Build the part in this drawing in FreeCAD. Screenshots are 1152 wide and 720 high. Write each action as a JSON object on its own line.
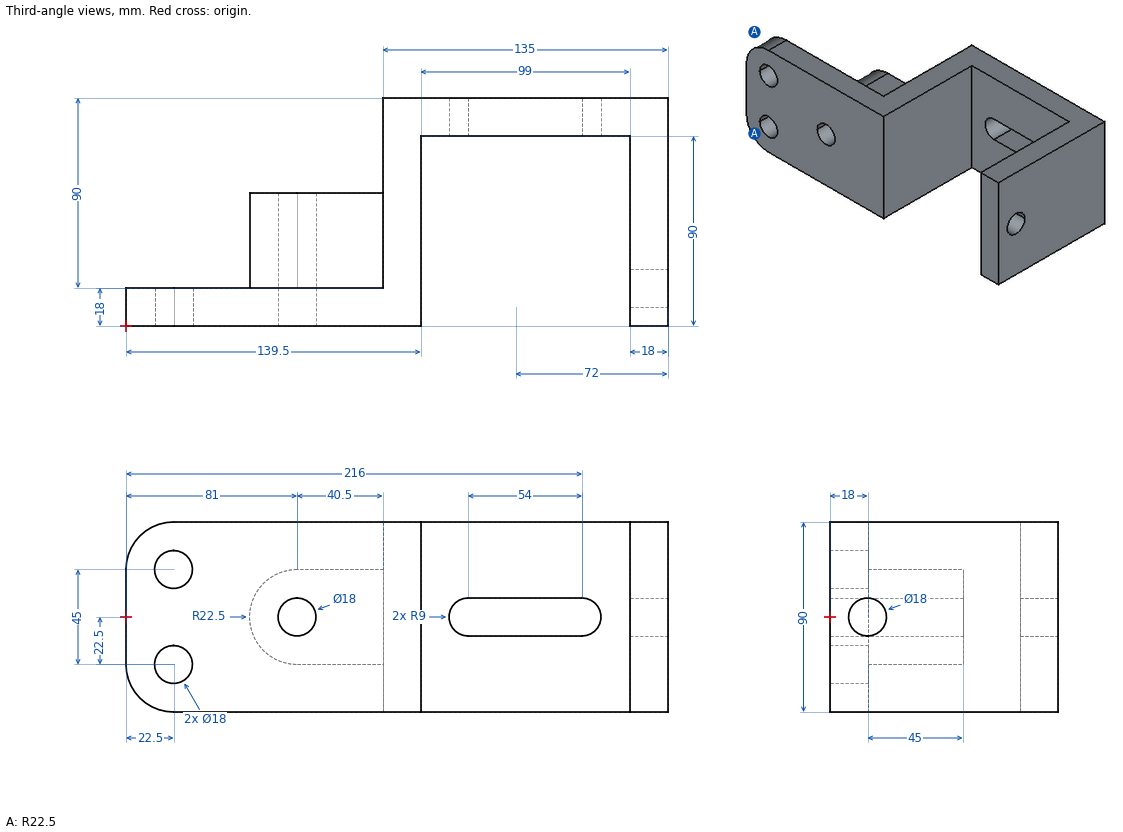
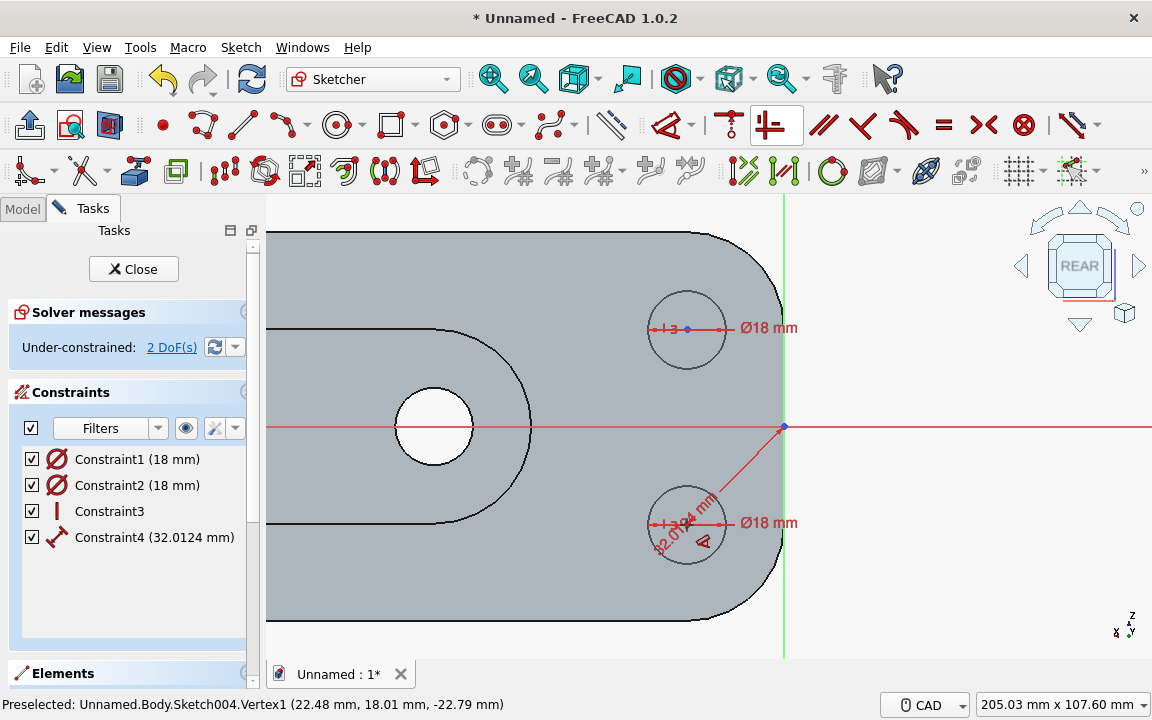
{"action": "left_click", "coordinate": [687, 330]}
{"action": "left_click", "coordinate": [653, 383]}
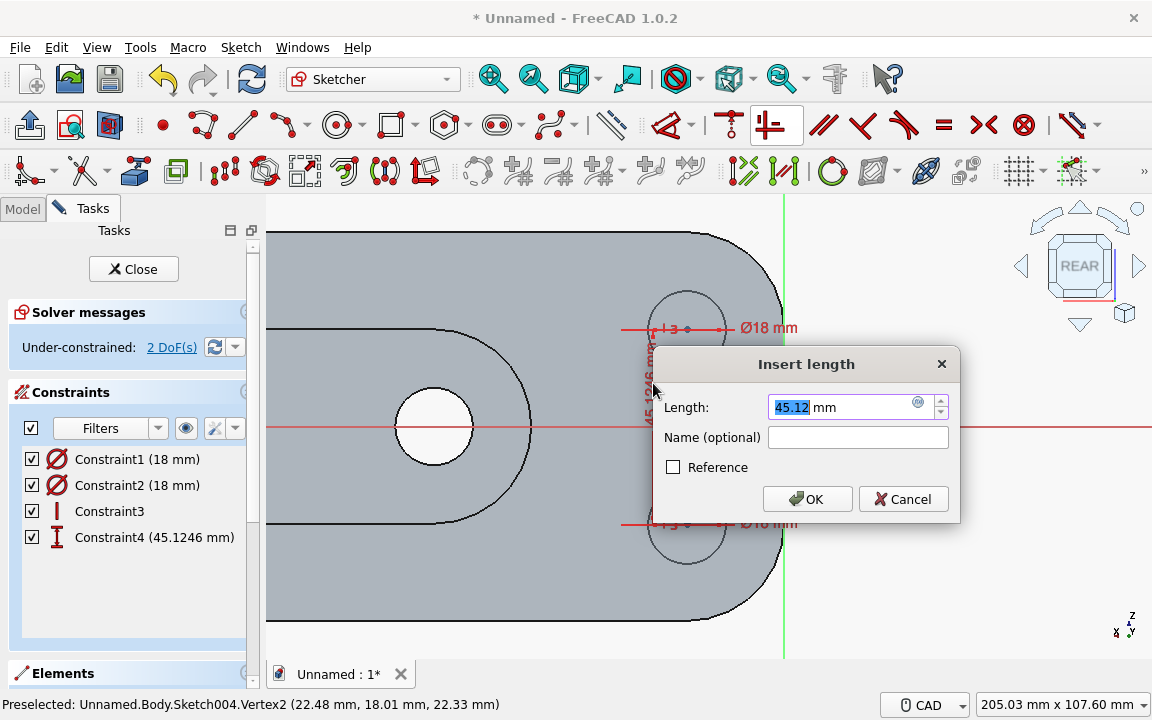
{"action": "type", "text": "45"}
{"action": "key", "text": "Return"}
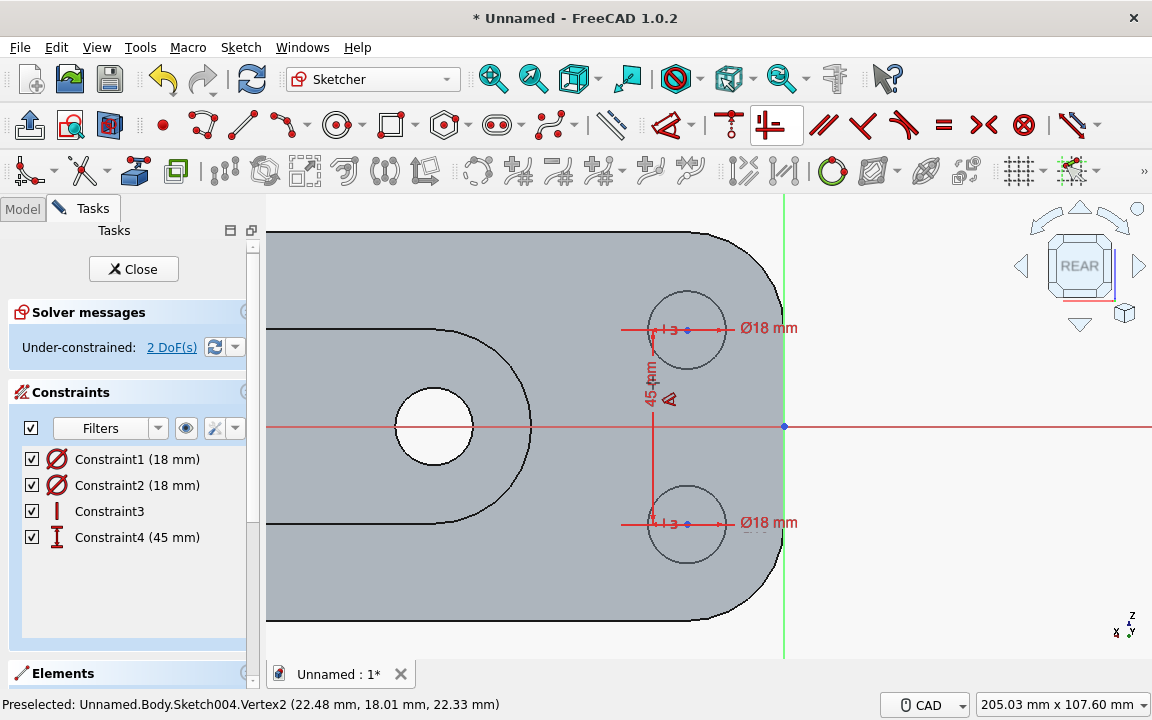
{"action": "left_click", "coordinate": [687, 525]}
{"action": "left_click", "coordinate": [736, 559]}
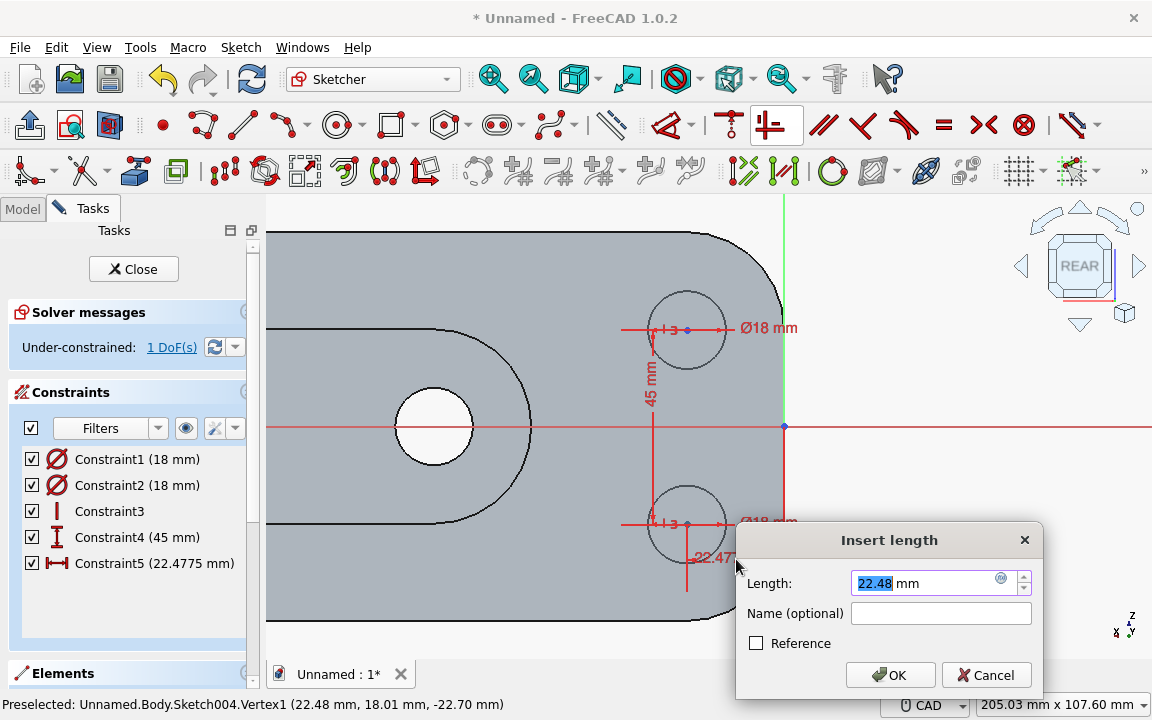
{"action": "type", "text": "22.5"}
{"action": "key", "text": "Return"}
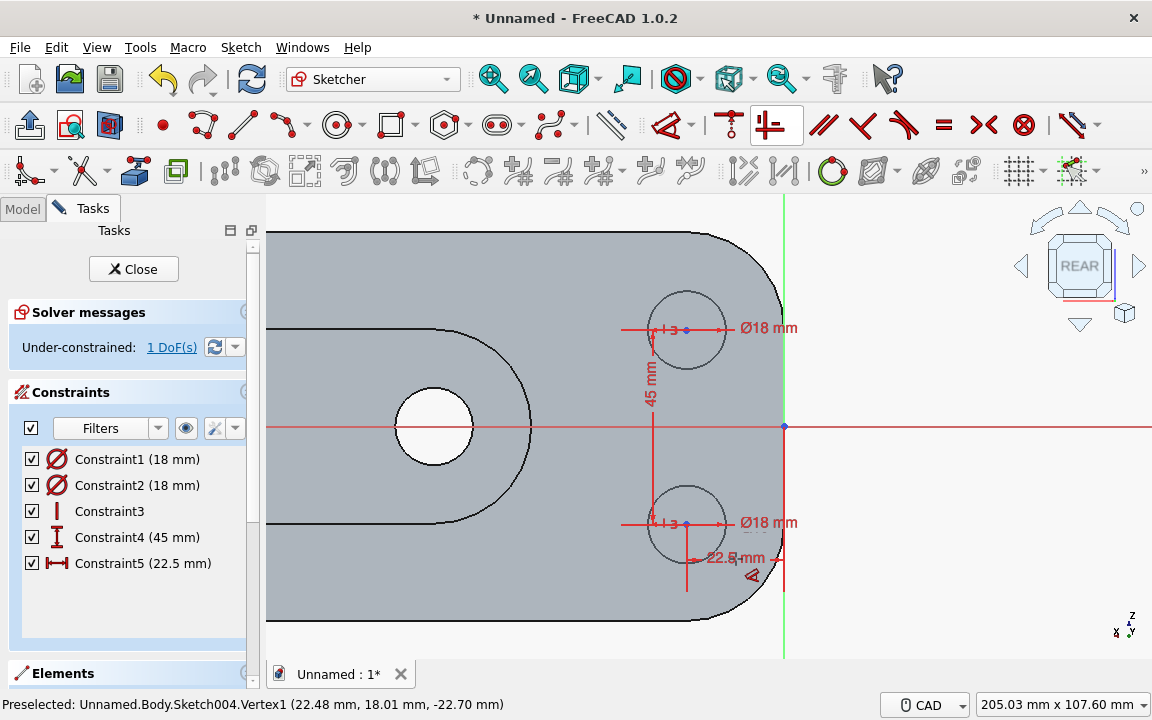
{"action": "left_click", "coordinate": [687, 525]}
{"action": "left_click", "coordinate": [818, 476]}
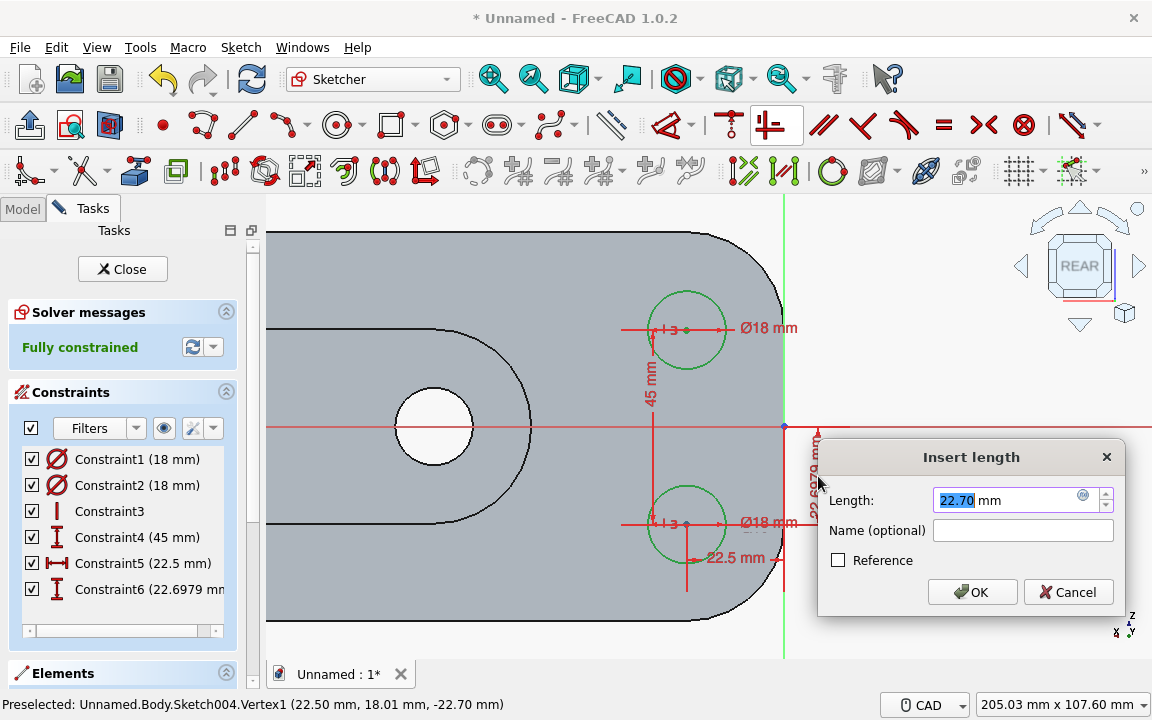
{"action": "type", "text": "22.5"}
{"action": "key", "text": "Return"}
{"action": "key", "text": "Escape"}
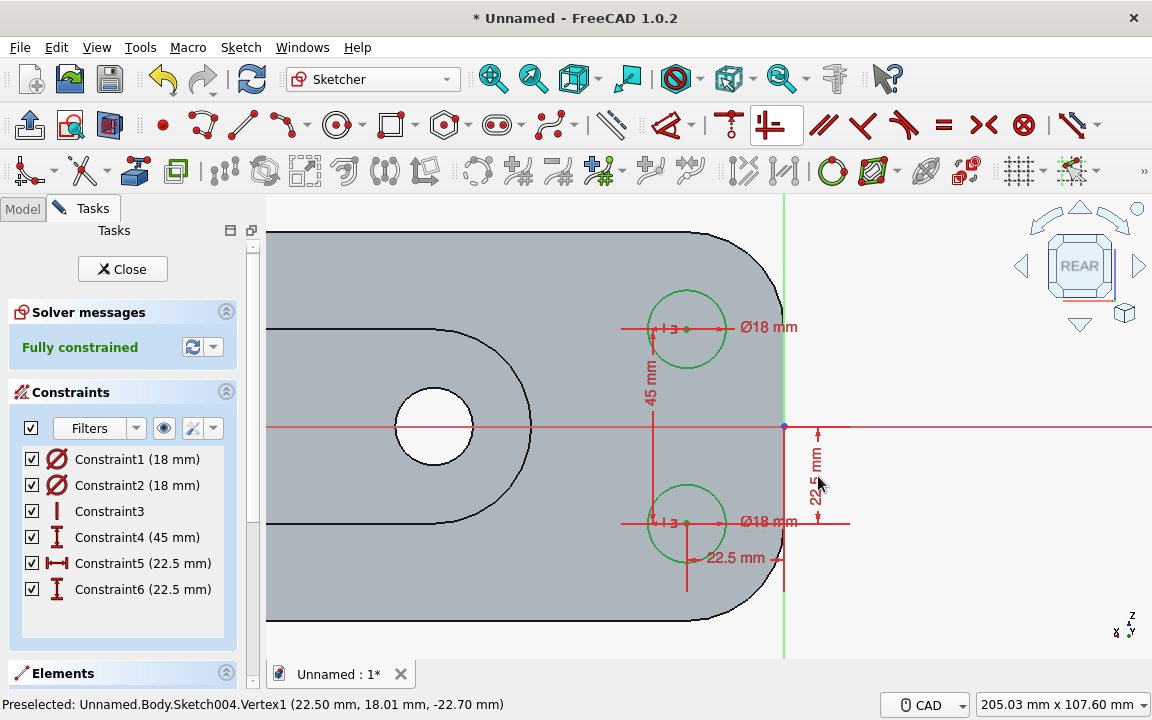
{"action": "left_click", "coordinate": [123, 269]}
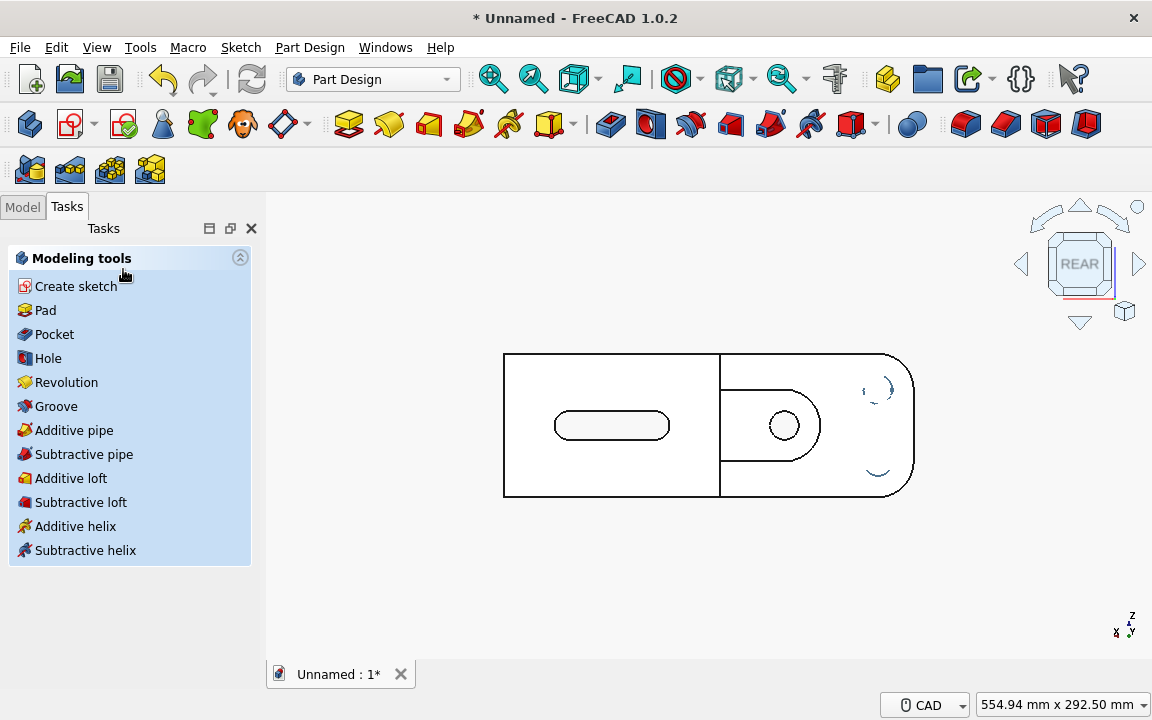
{"action": "left_click", "coordinate": [612, 124]}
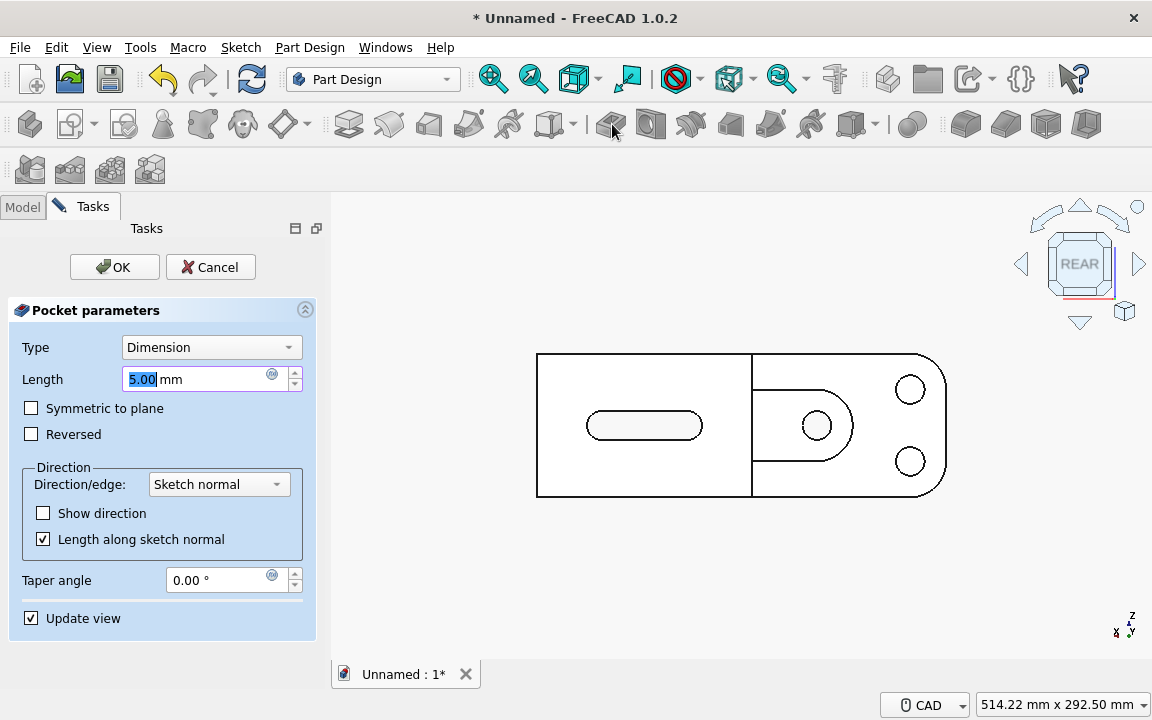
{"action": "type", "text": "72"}
{"action": "key", "text": "Tab"}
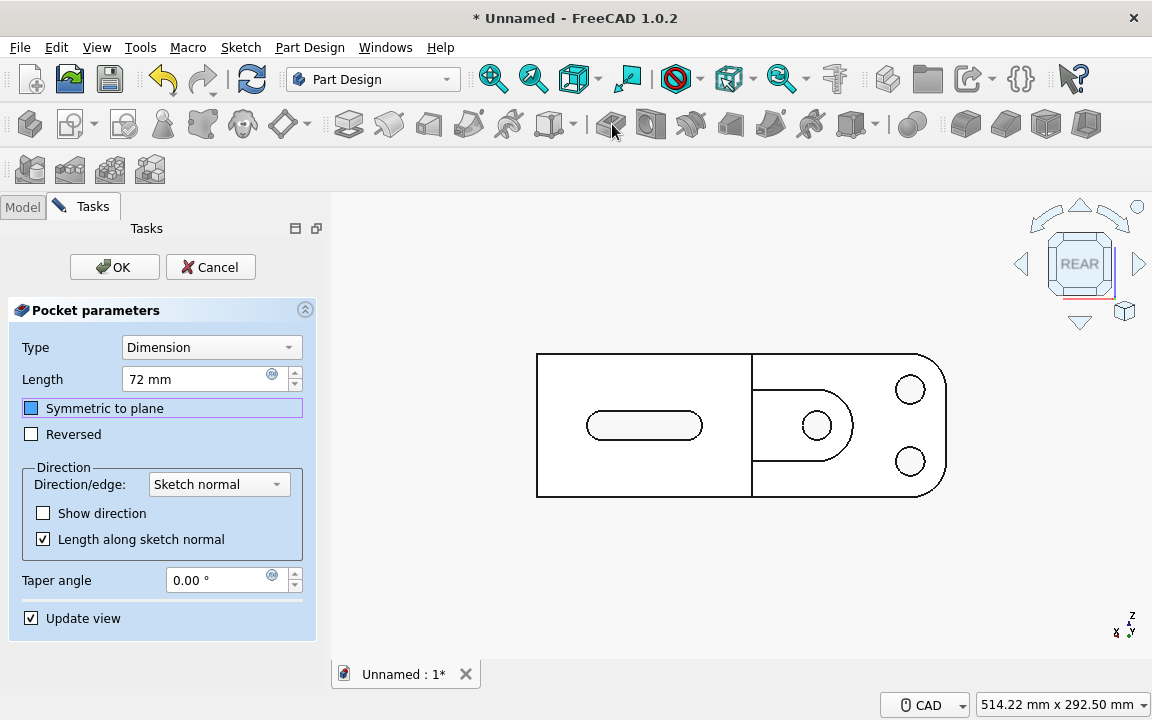
{"action": "left_click", "coordinate": [115, 267]}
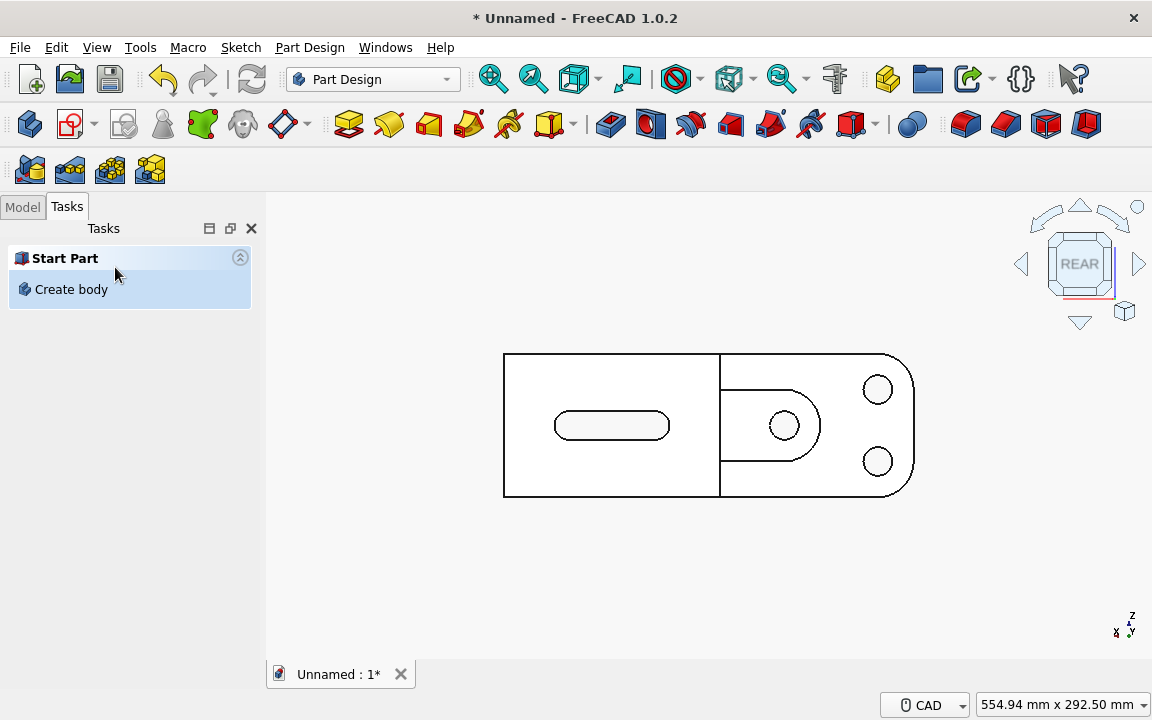
{"action": "key", "text": "0"}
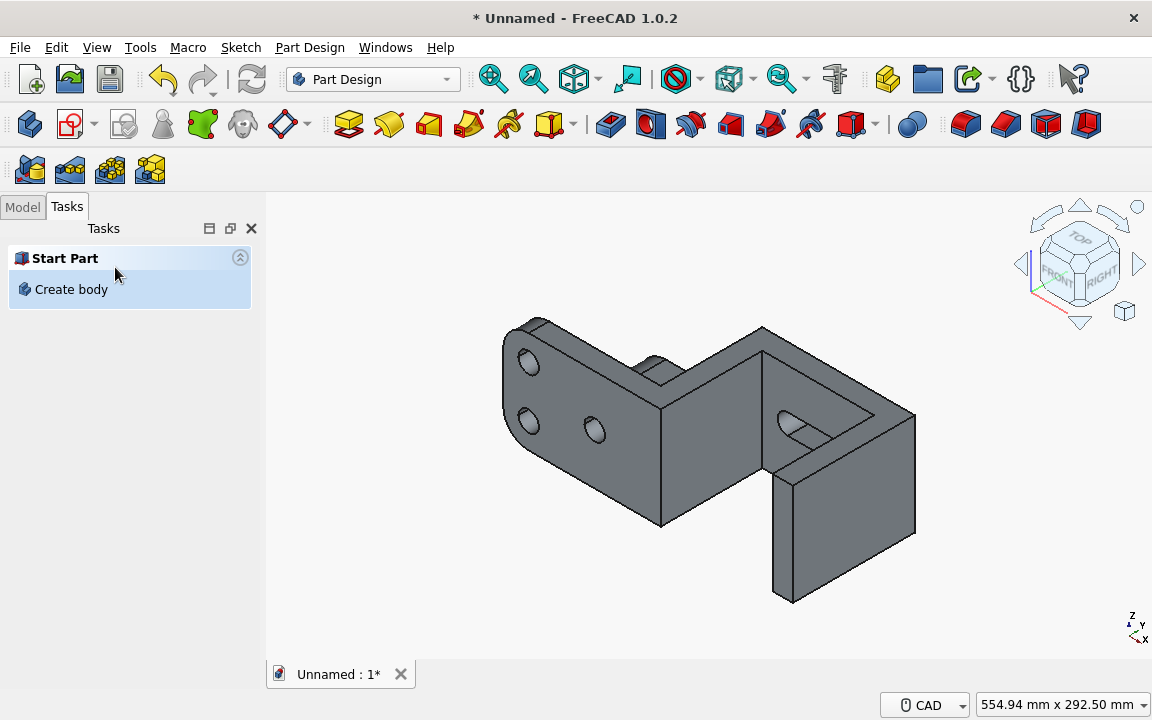
{"action": "left_click", "coordinate": [854, 508]}